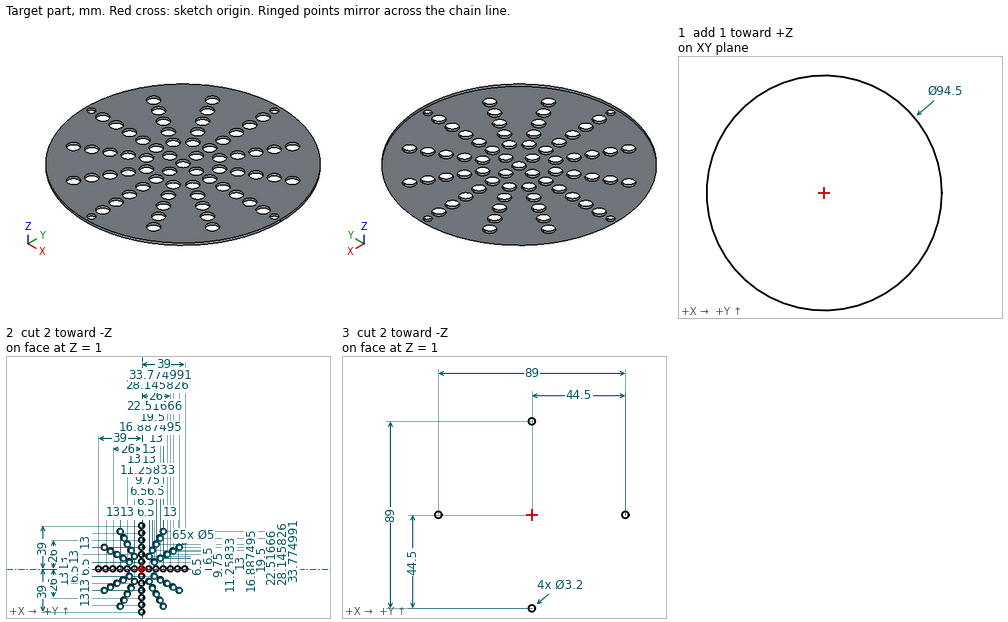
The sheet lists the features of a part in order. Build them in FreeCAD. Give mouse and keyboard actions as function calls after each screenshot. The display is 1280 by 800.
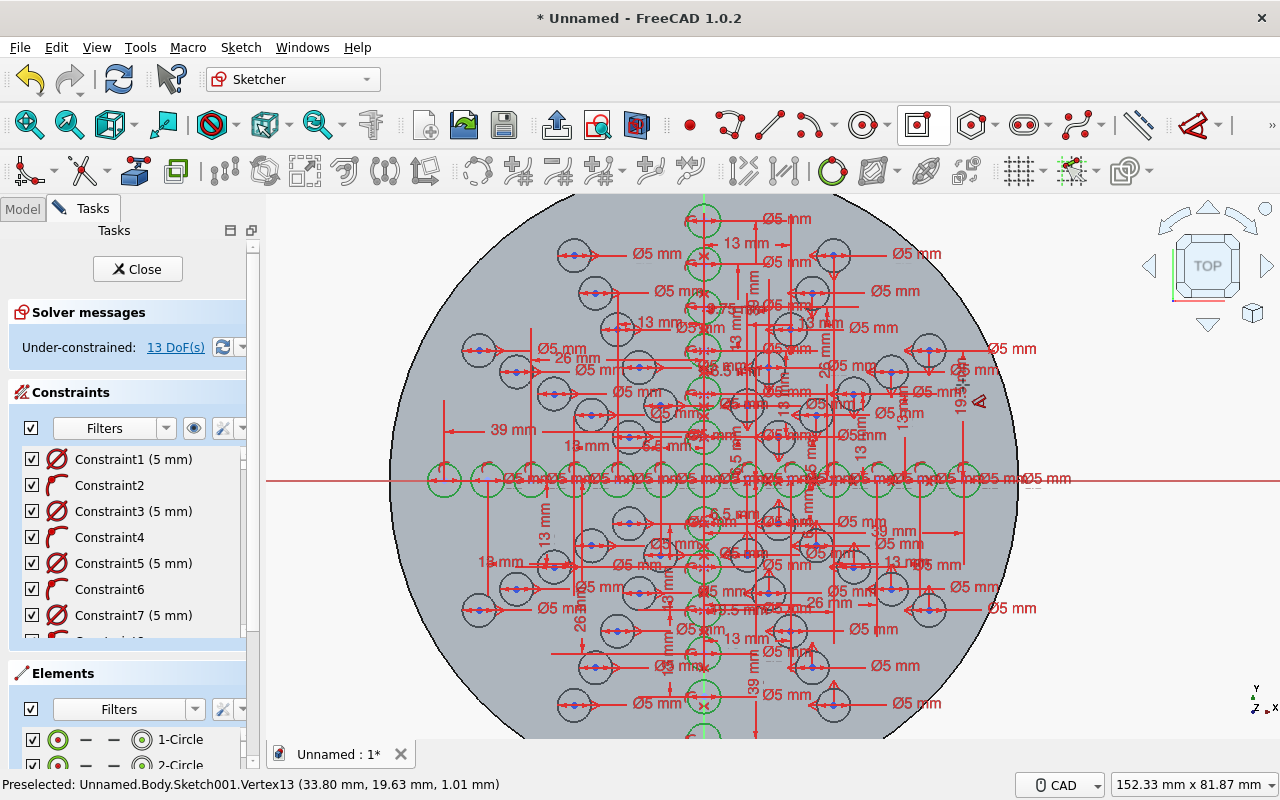
click(816, 415)
click(946, 448)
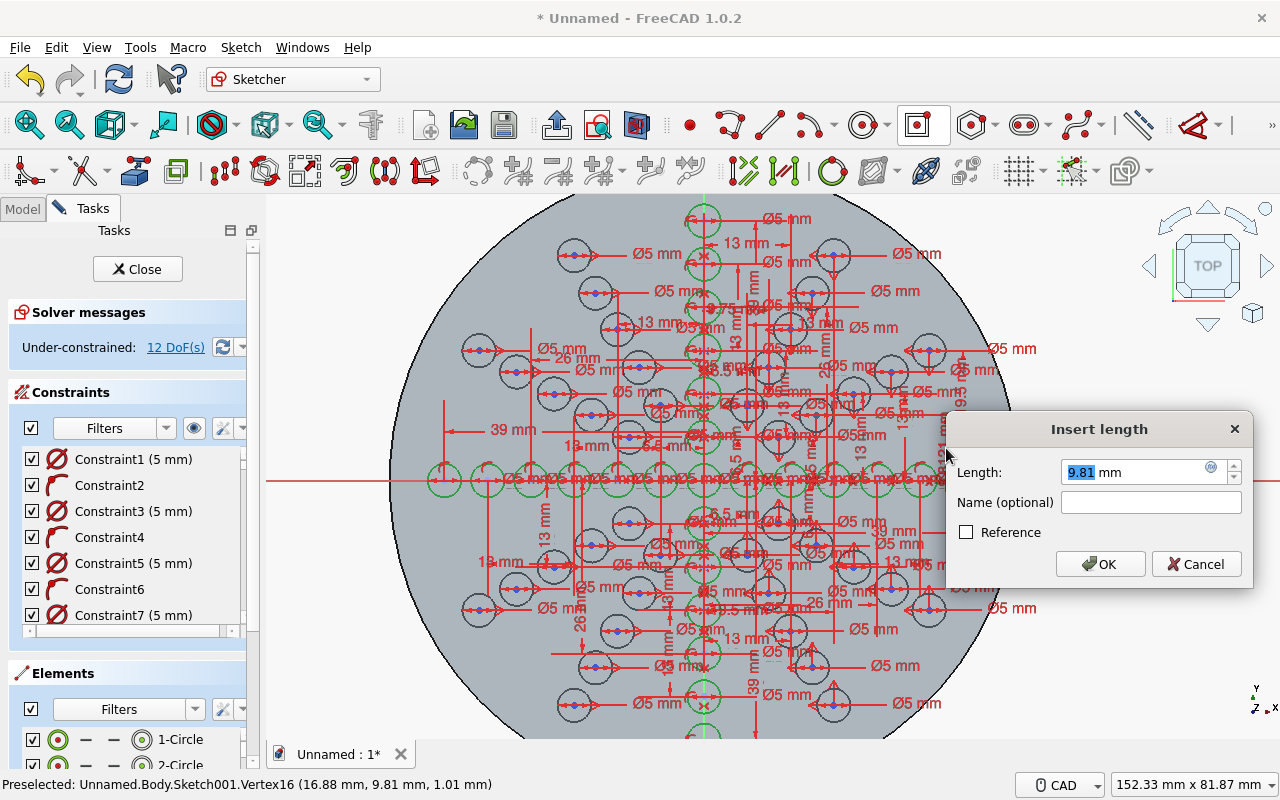
text(9.75)
key(Return)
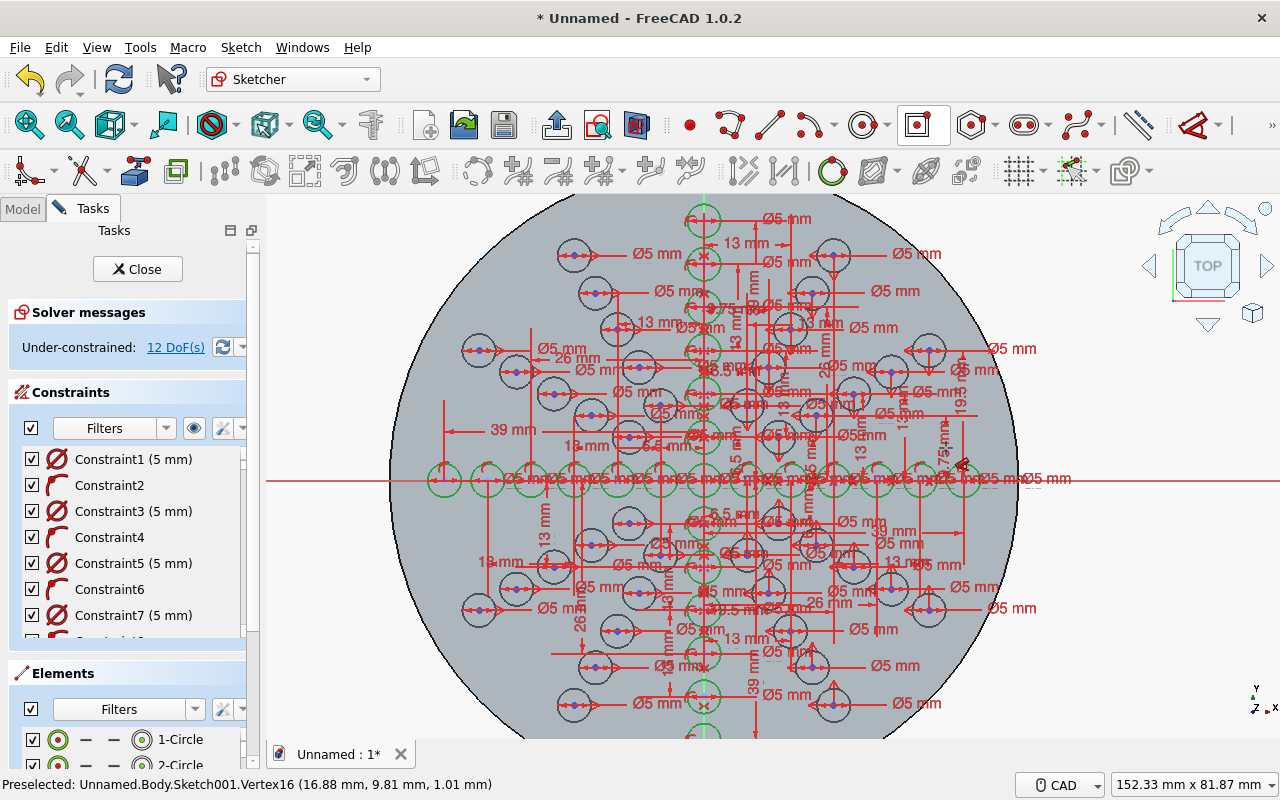
click(812, 293)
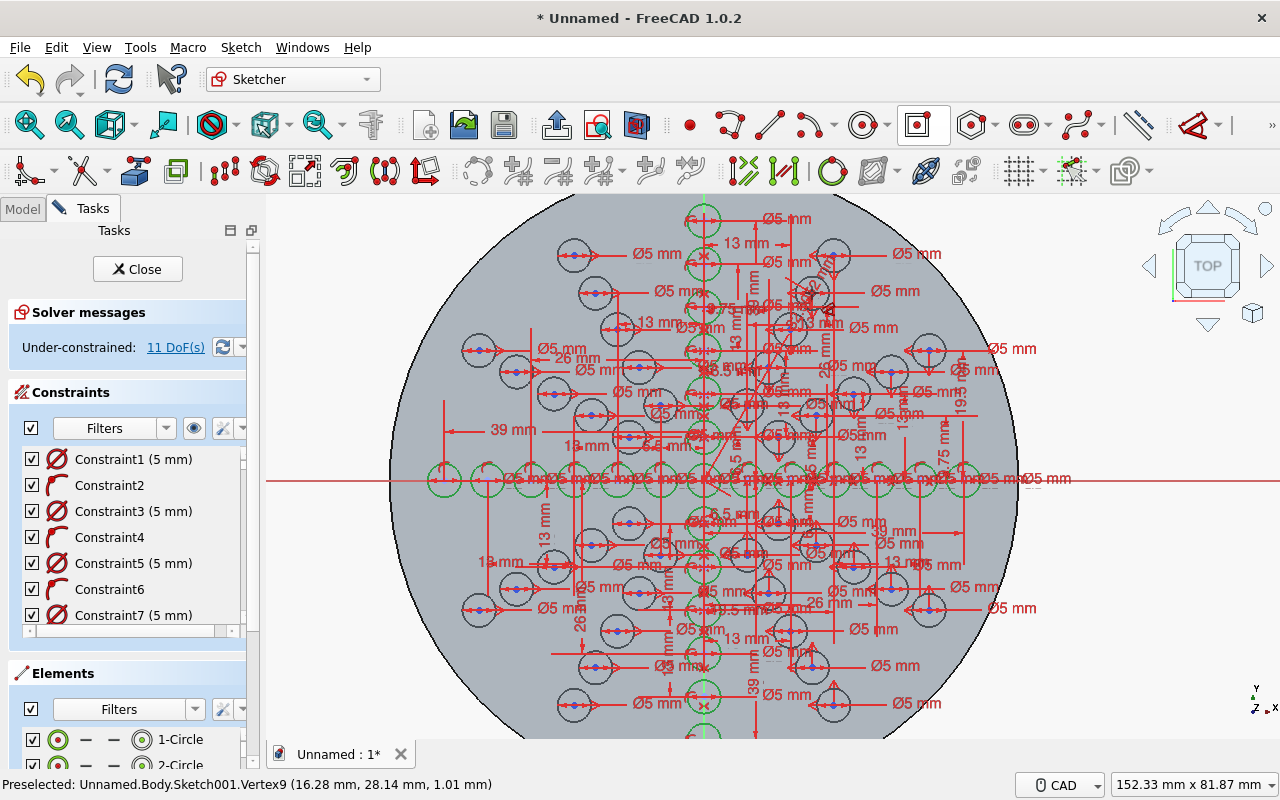
click(769, 368)
click(791, 259)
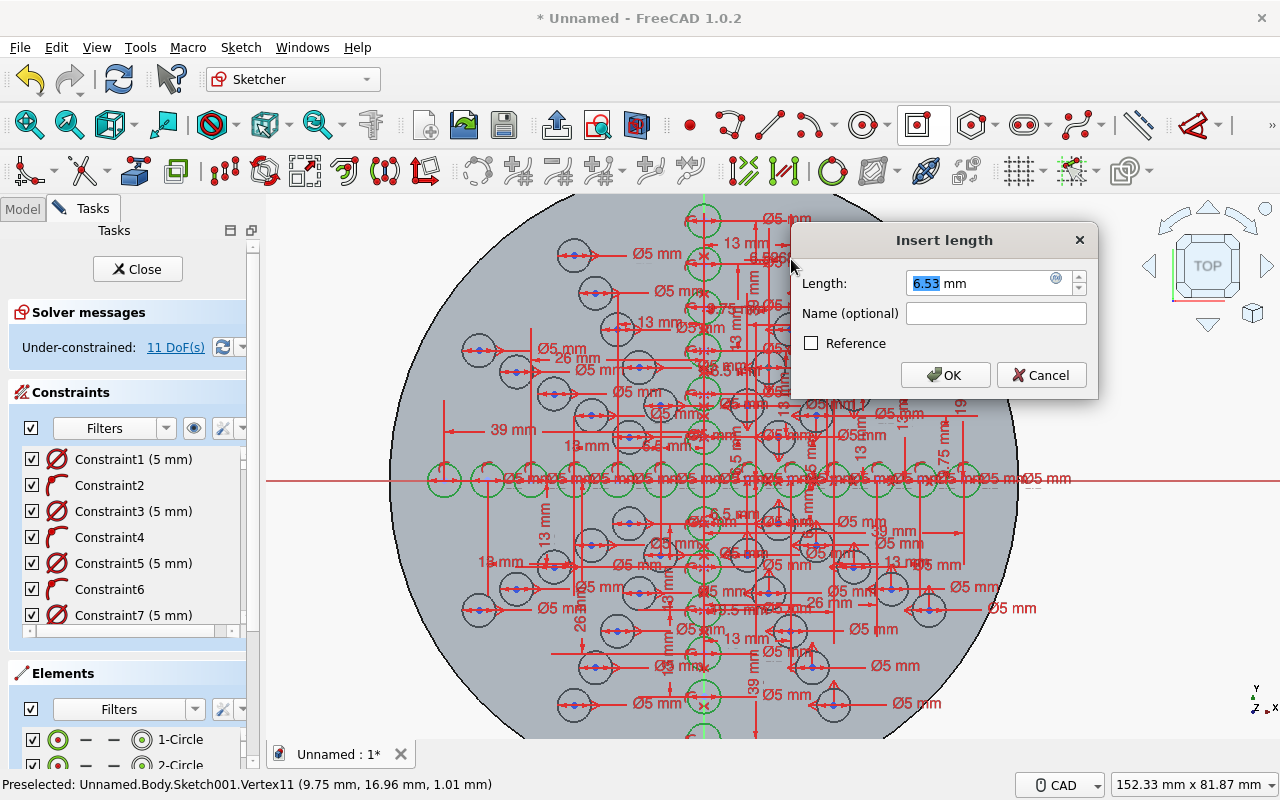
text(6.5)
key(Return)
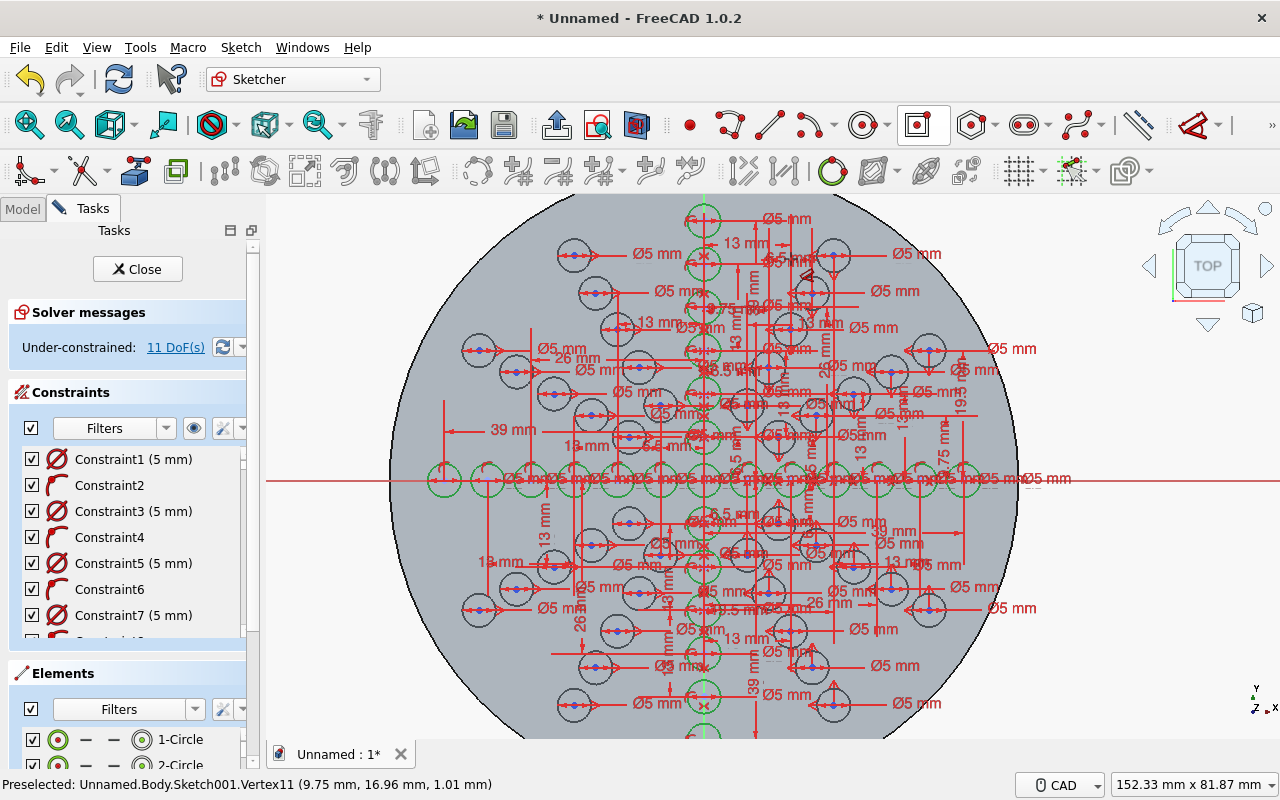
click(892, 372)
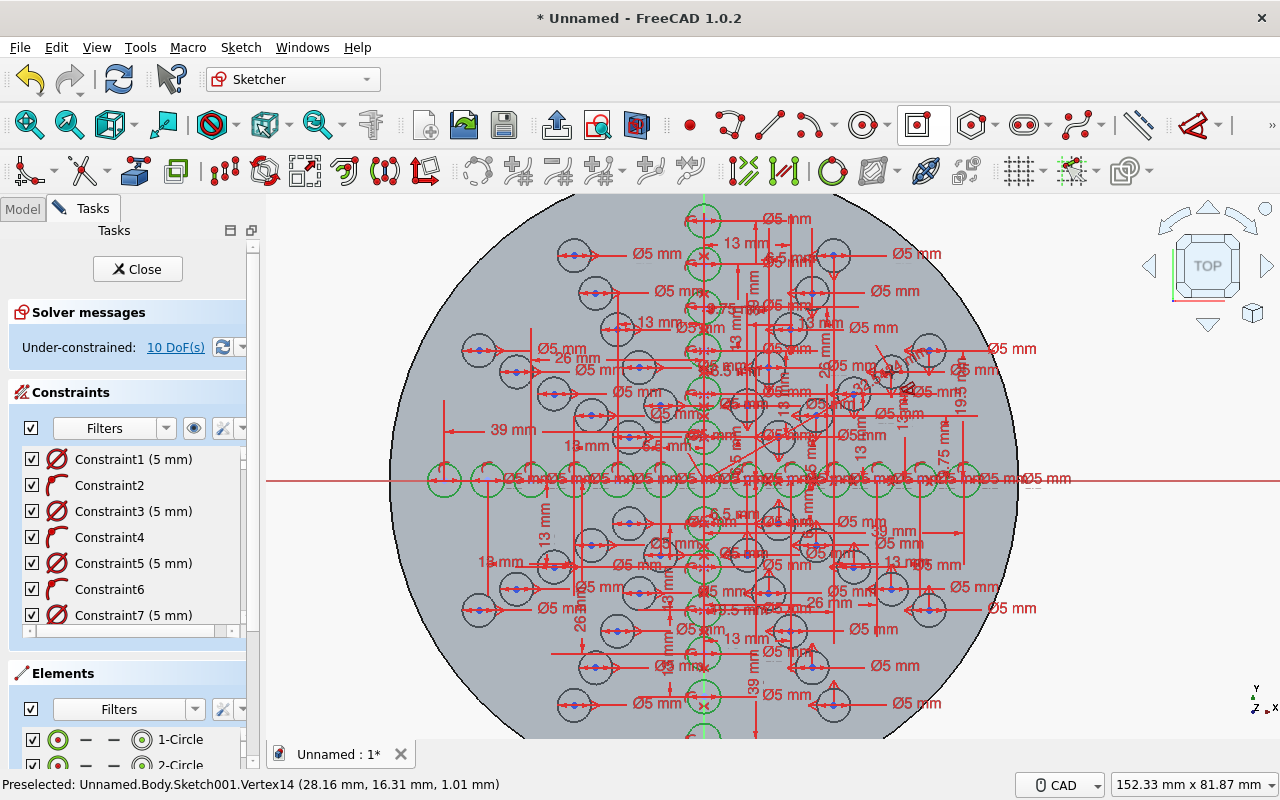
click(816, 416)
click(998, 409)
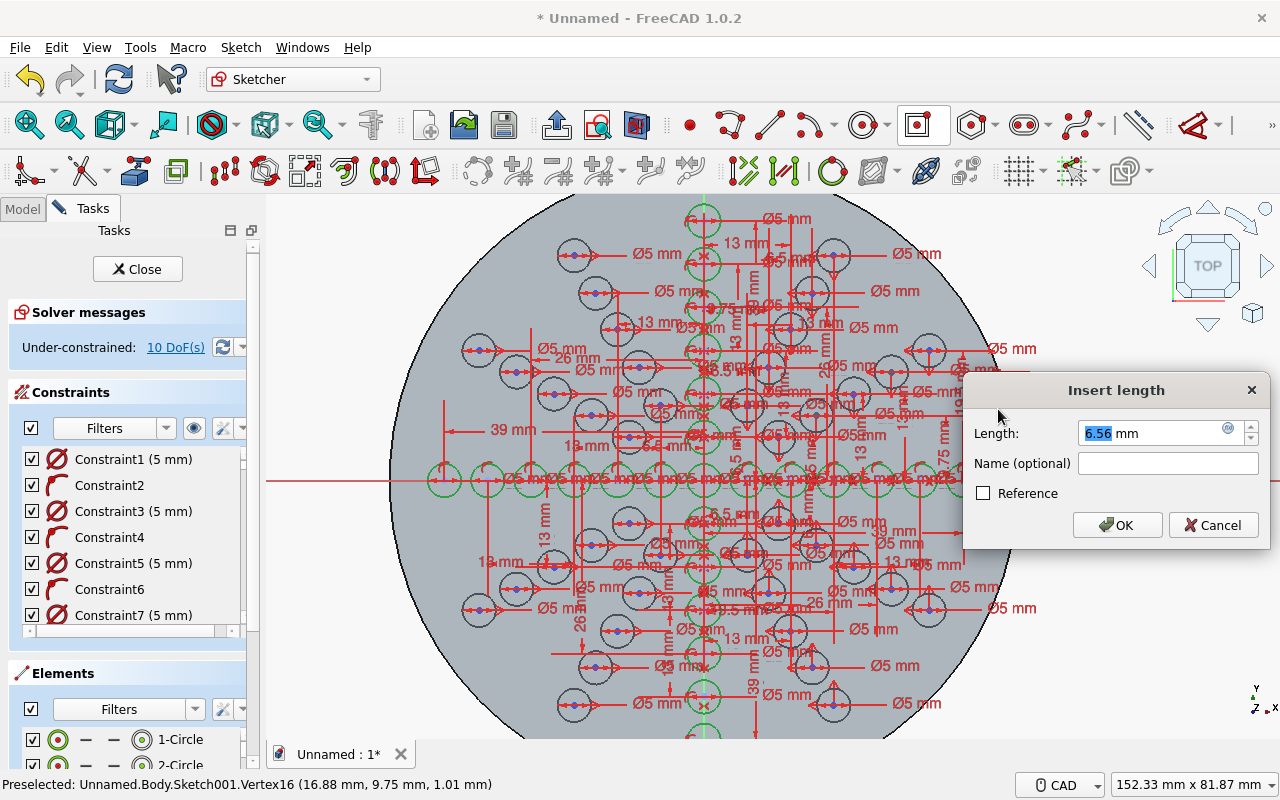
text(6.5)
key(Return)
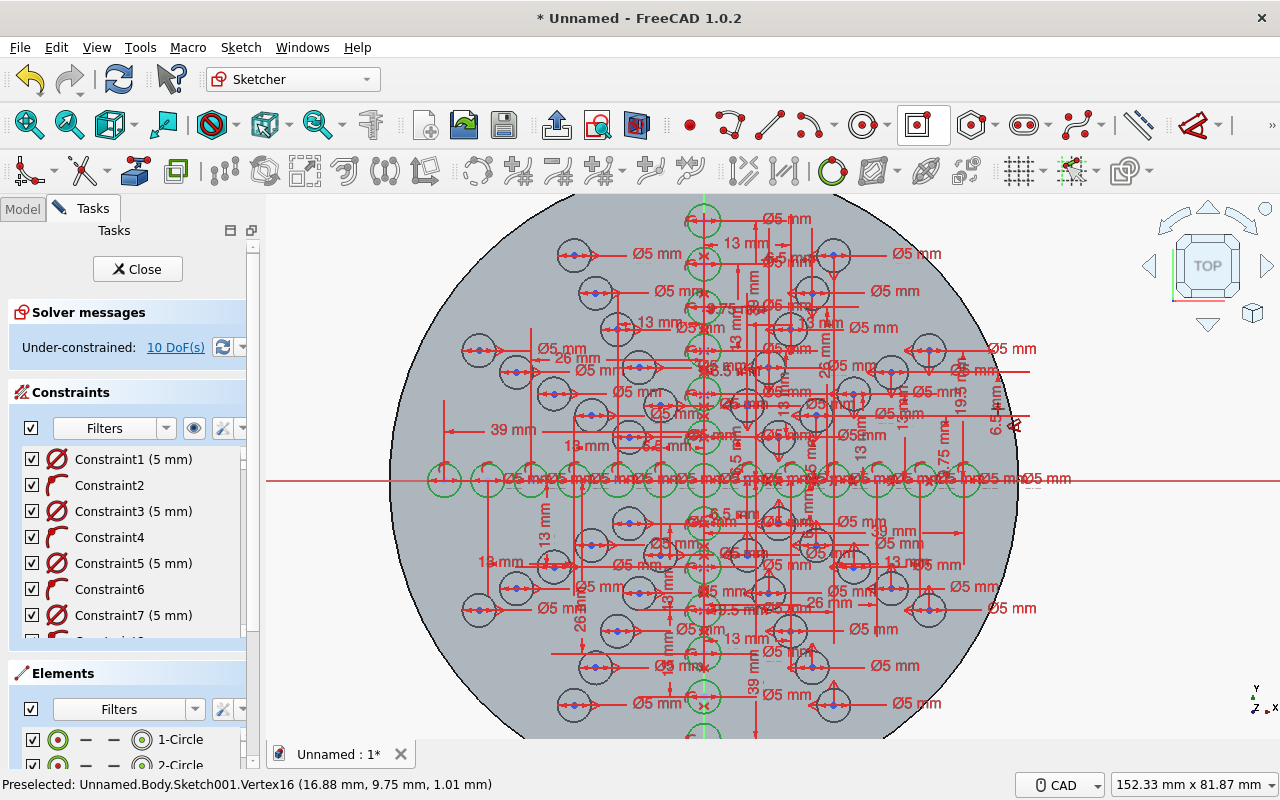
click(791, 330)
click(622, 405)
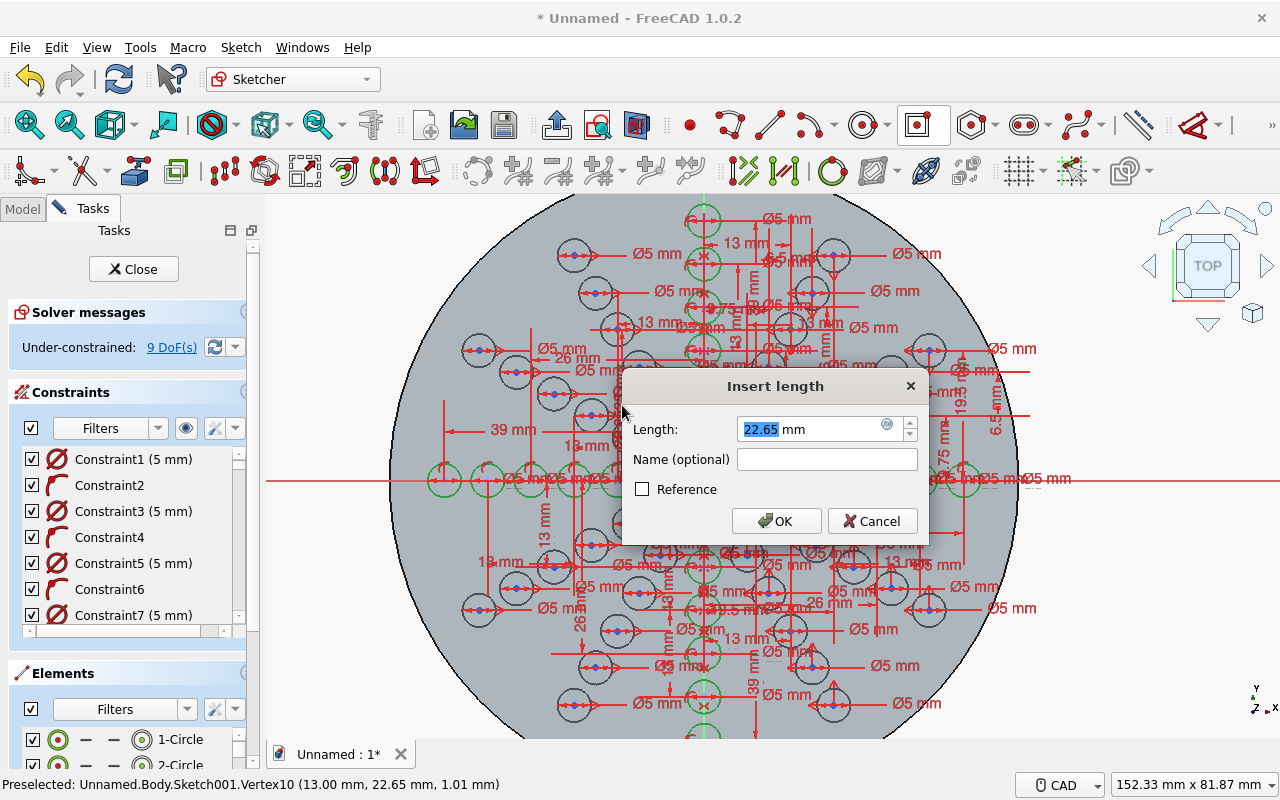
text(22.51666)
key(Return)